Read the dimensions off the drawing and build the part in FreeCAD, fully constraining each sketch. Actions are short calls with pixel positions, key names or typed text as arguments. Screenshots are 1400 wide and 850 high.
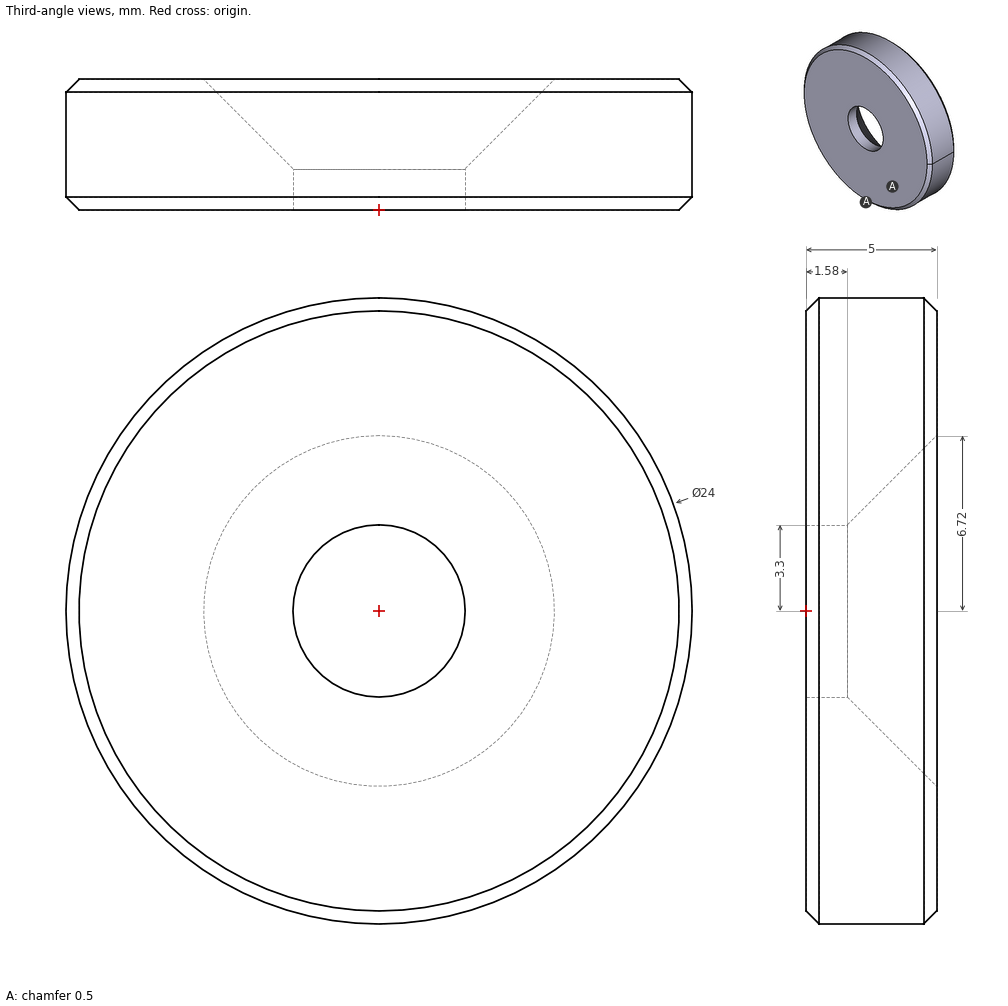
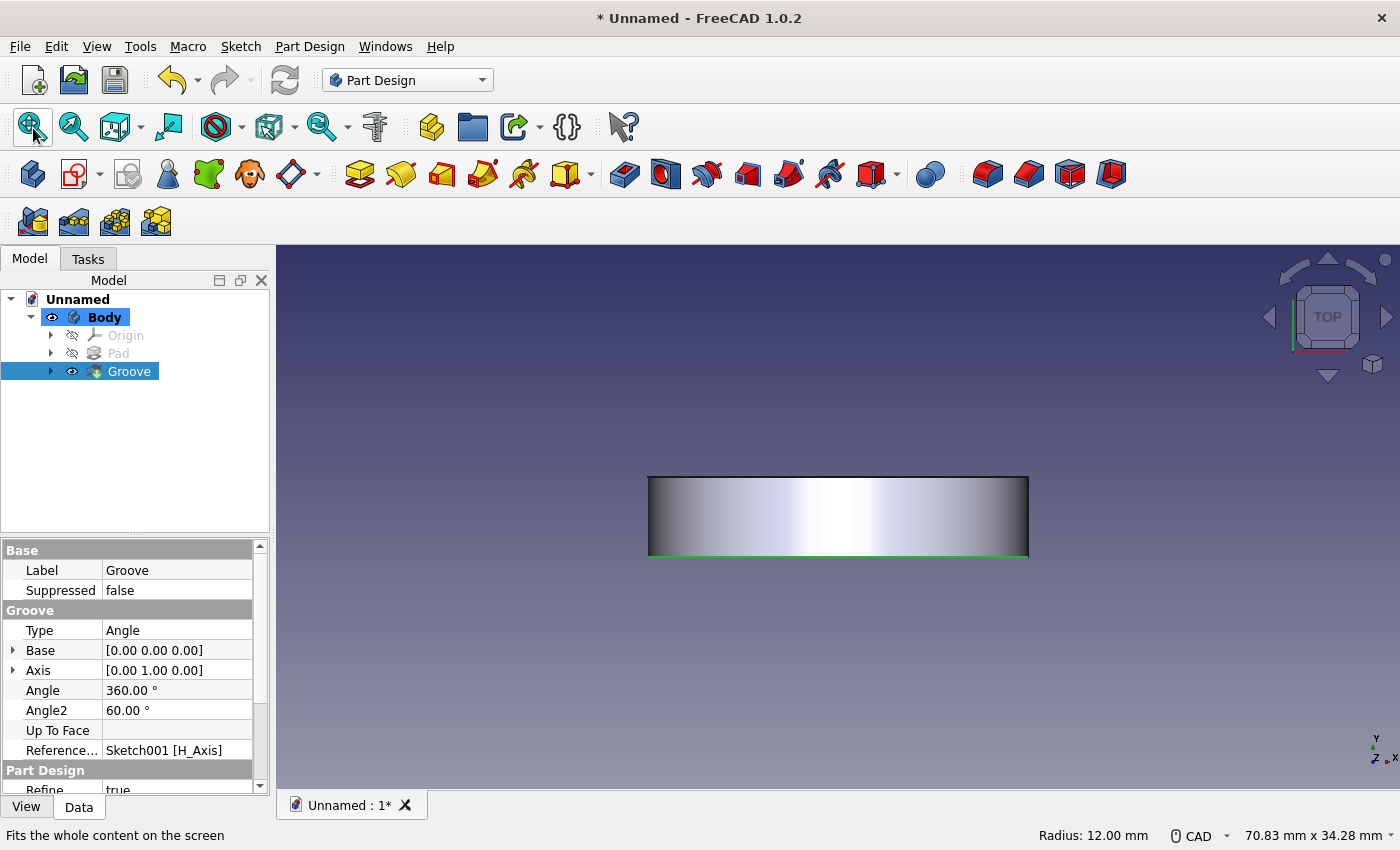
click(684, 476, ctrl)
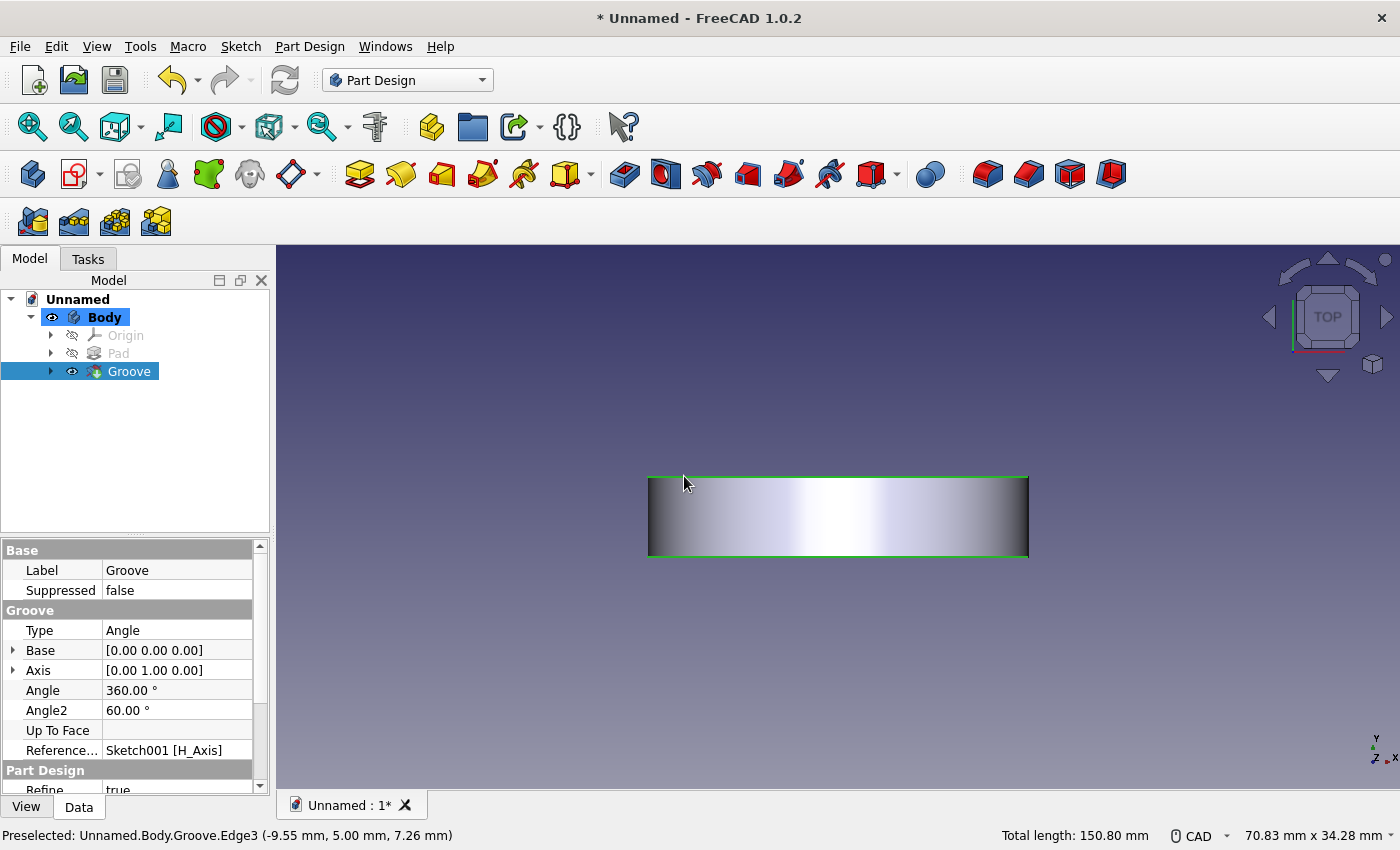
click(1029, 174)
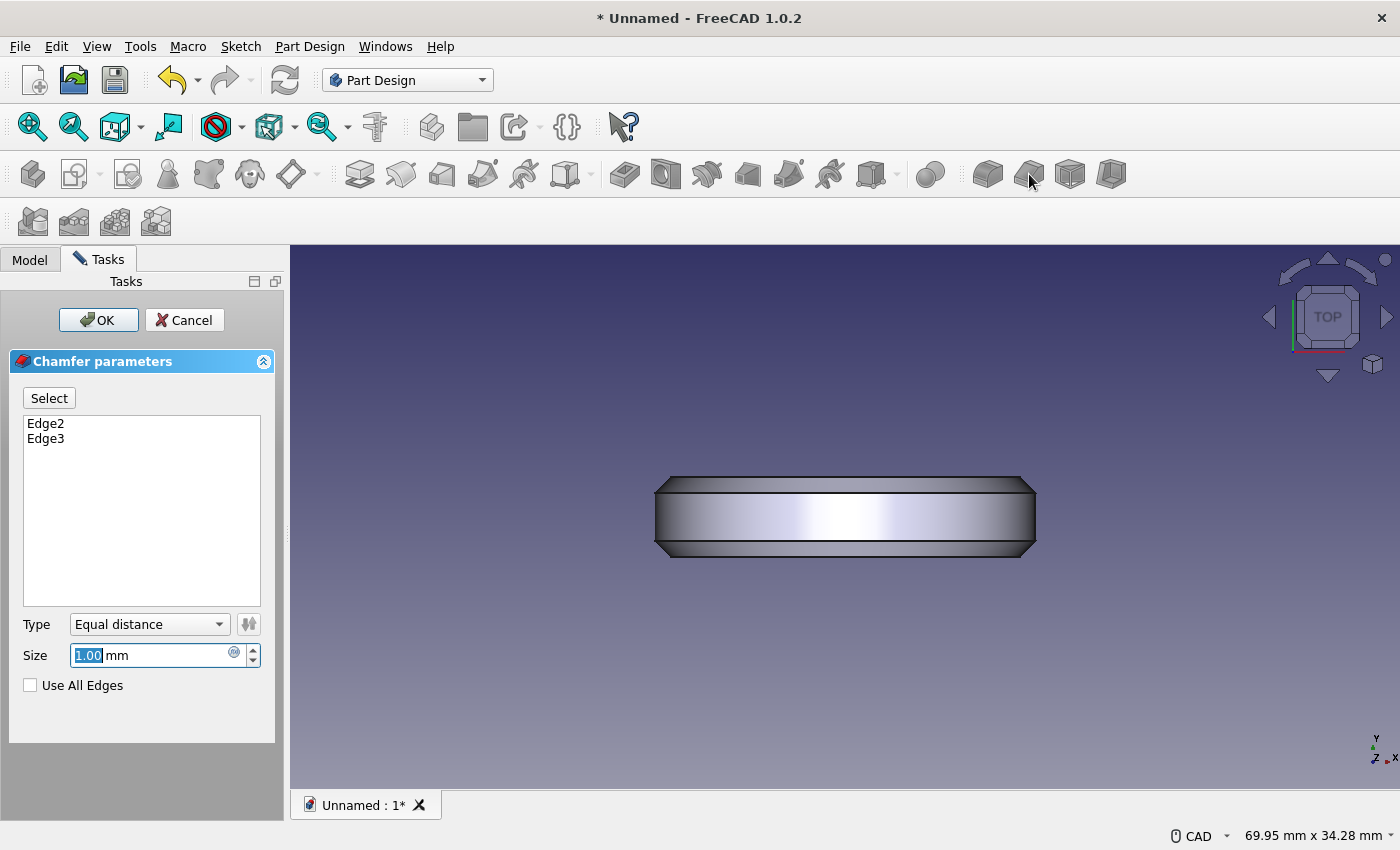
text(0.5)
key(Tab)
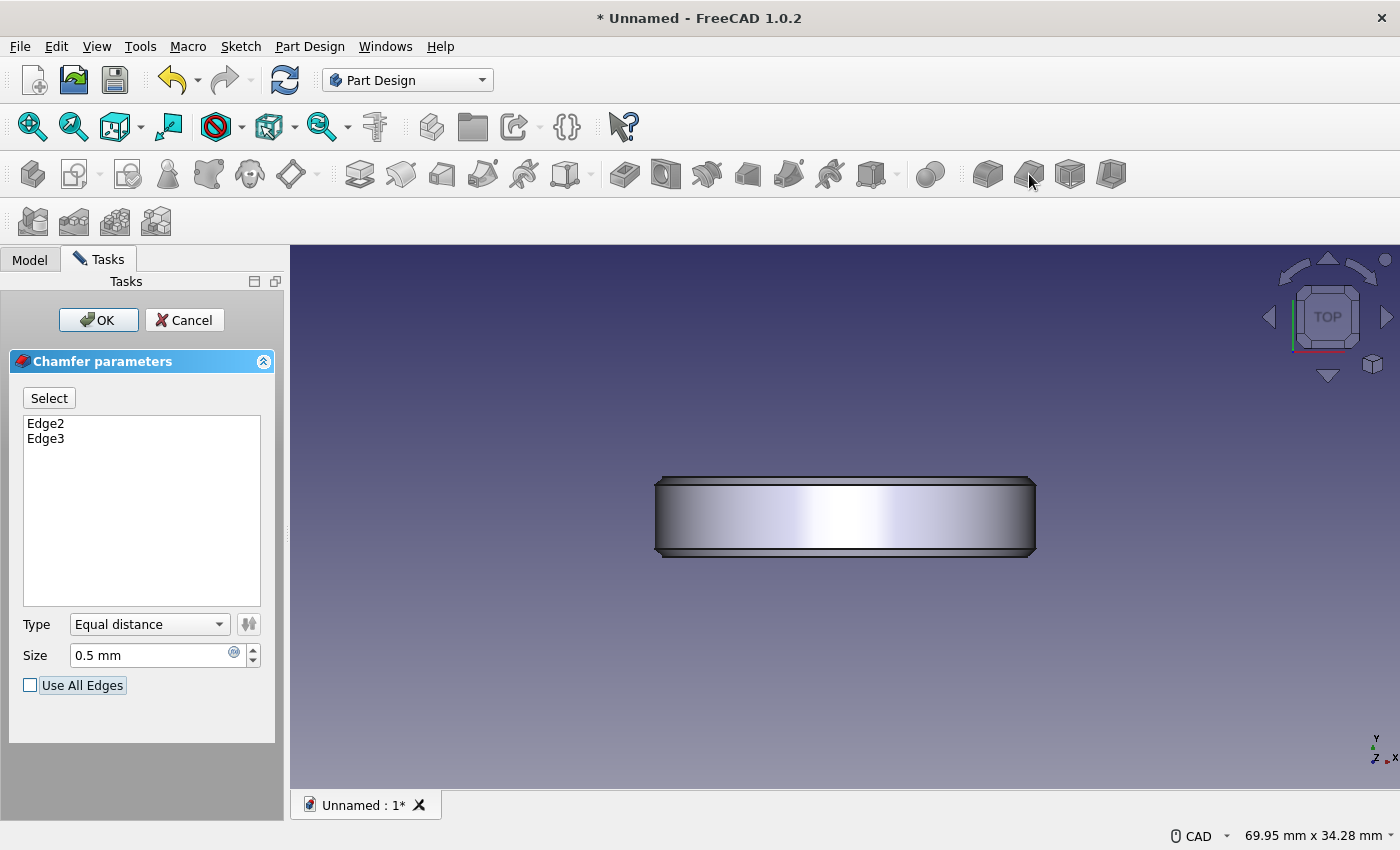
click(99, 320)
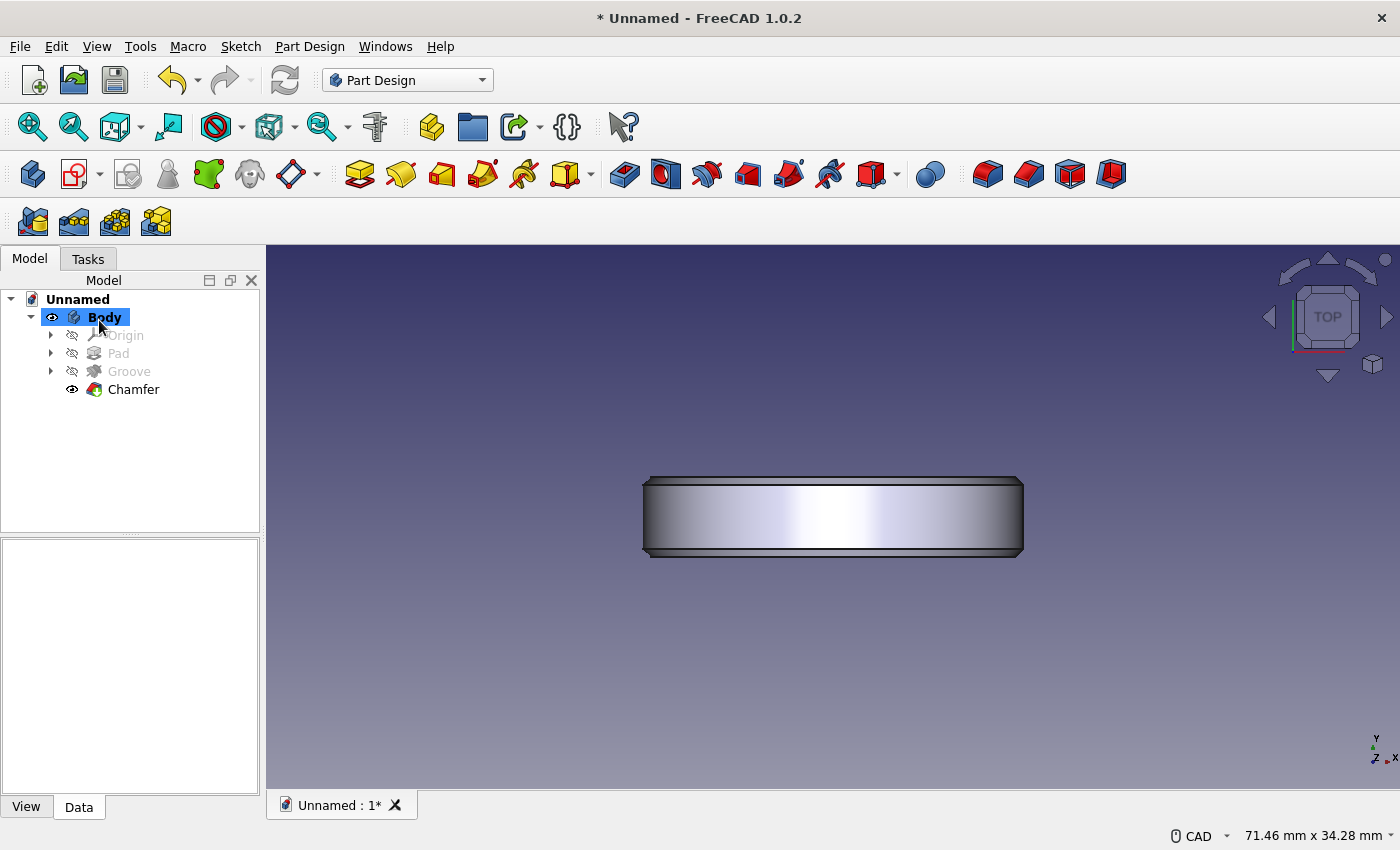
key(0)